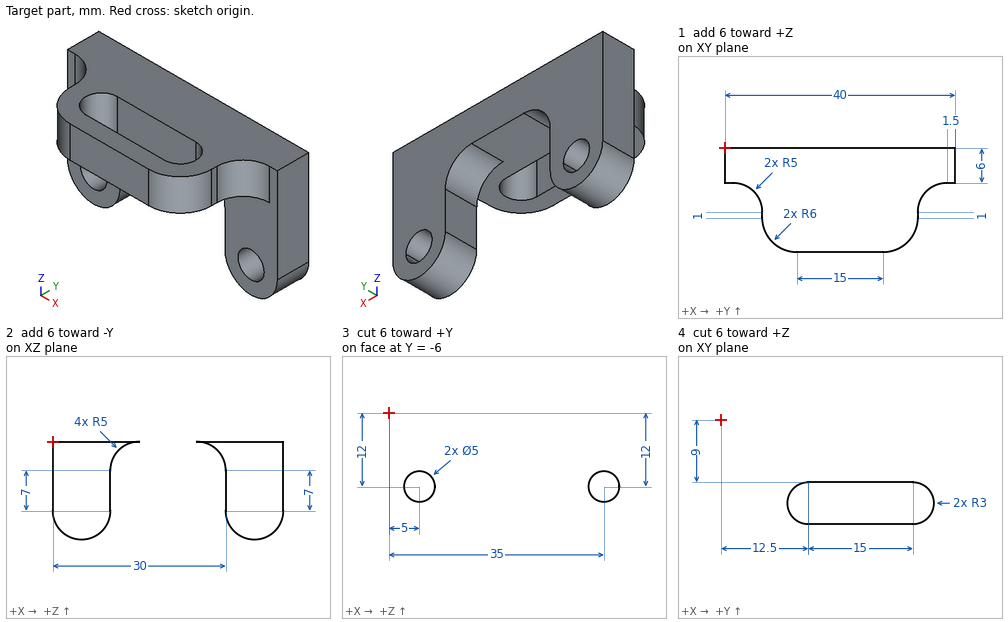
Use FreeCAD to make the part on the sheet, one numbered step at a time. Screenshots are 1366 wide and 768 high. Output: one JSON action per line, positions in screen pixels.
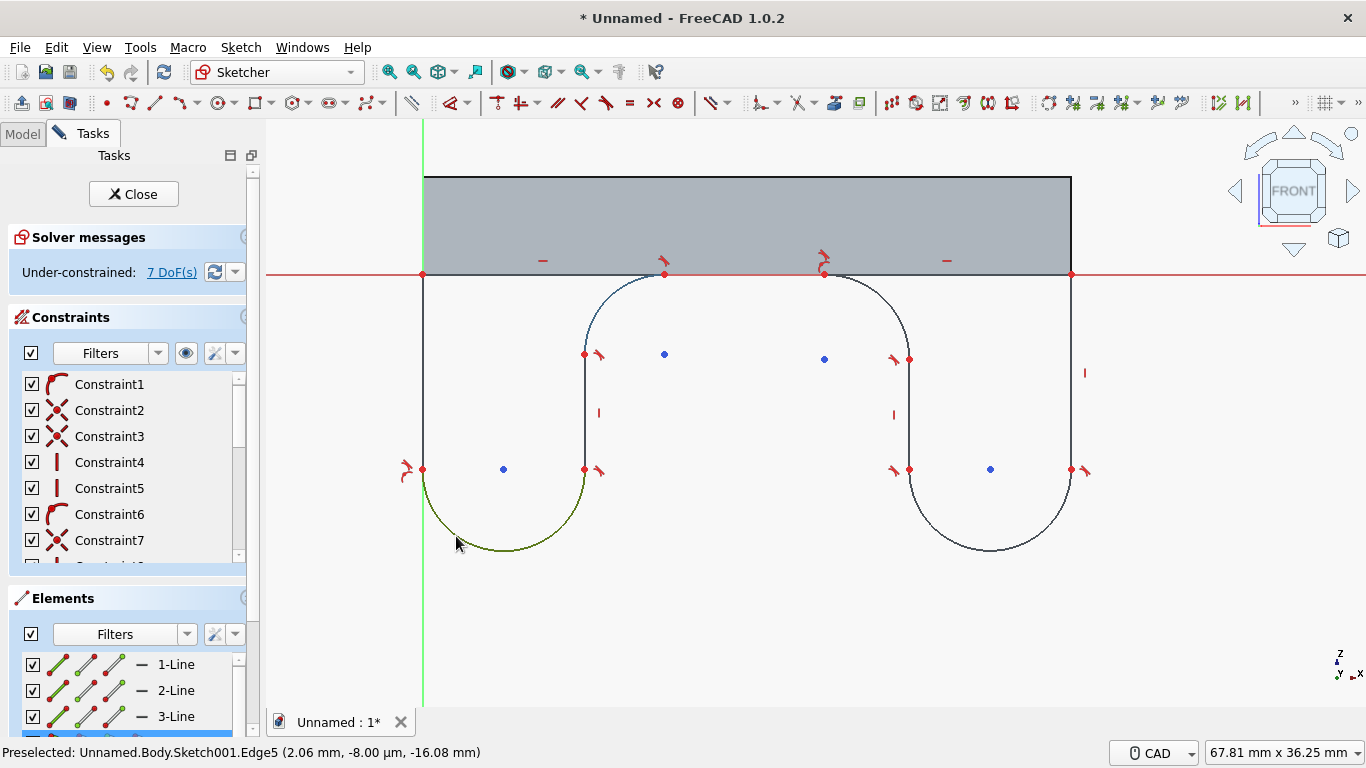
{"action": "left_click", "coordinate": [900, 321]}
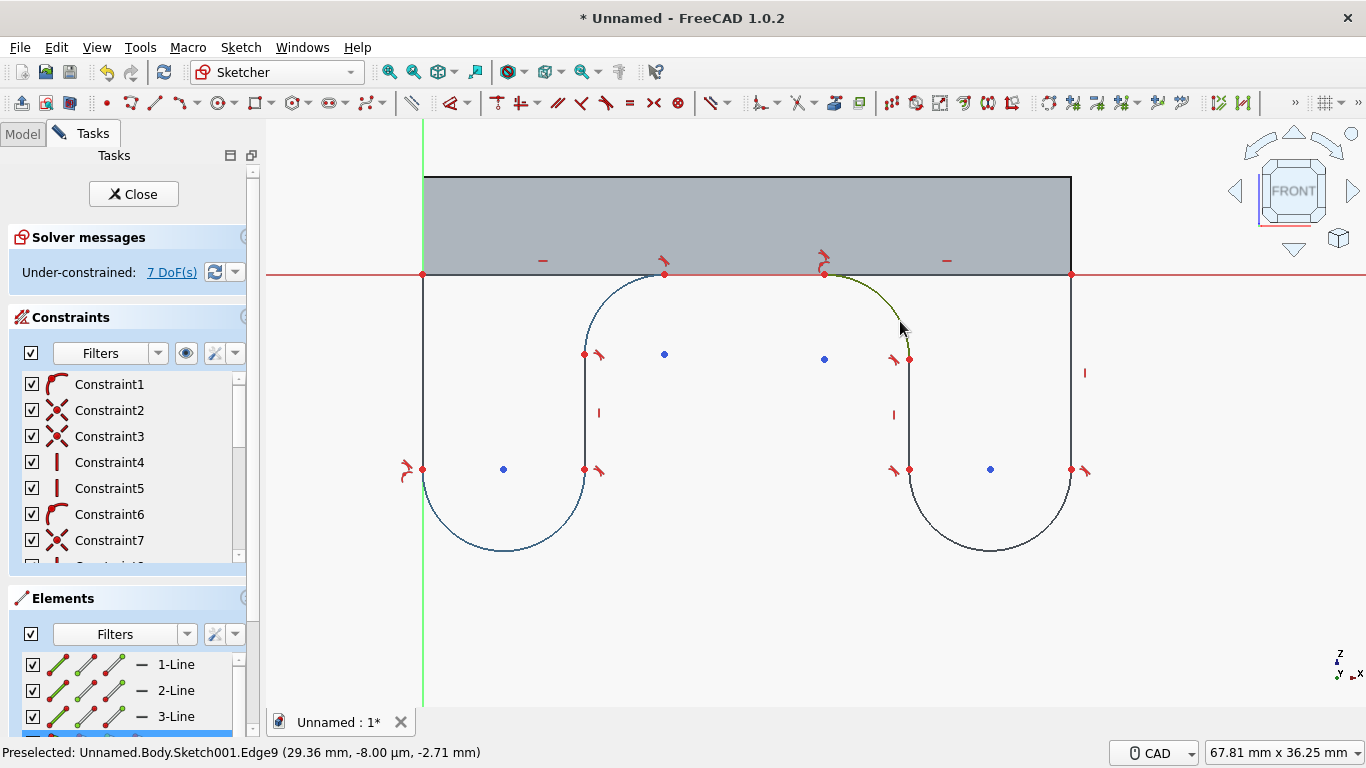
{"action": "left_click", "coordinate": [943, 535]}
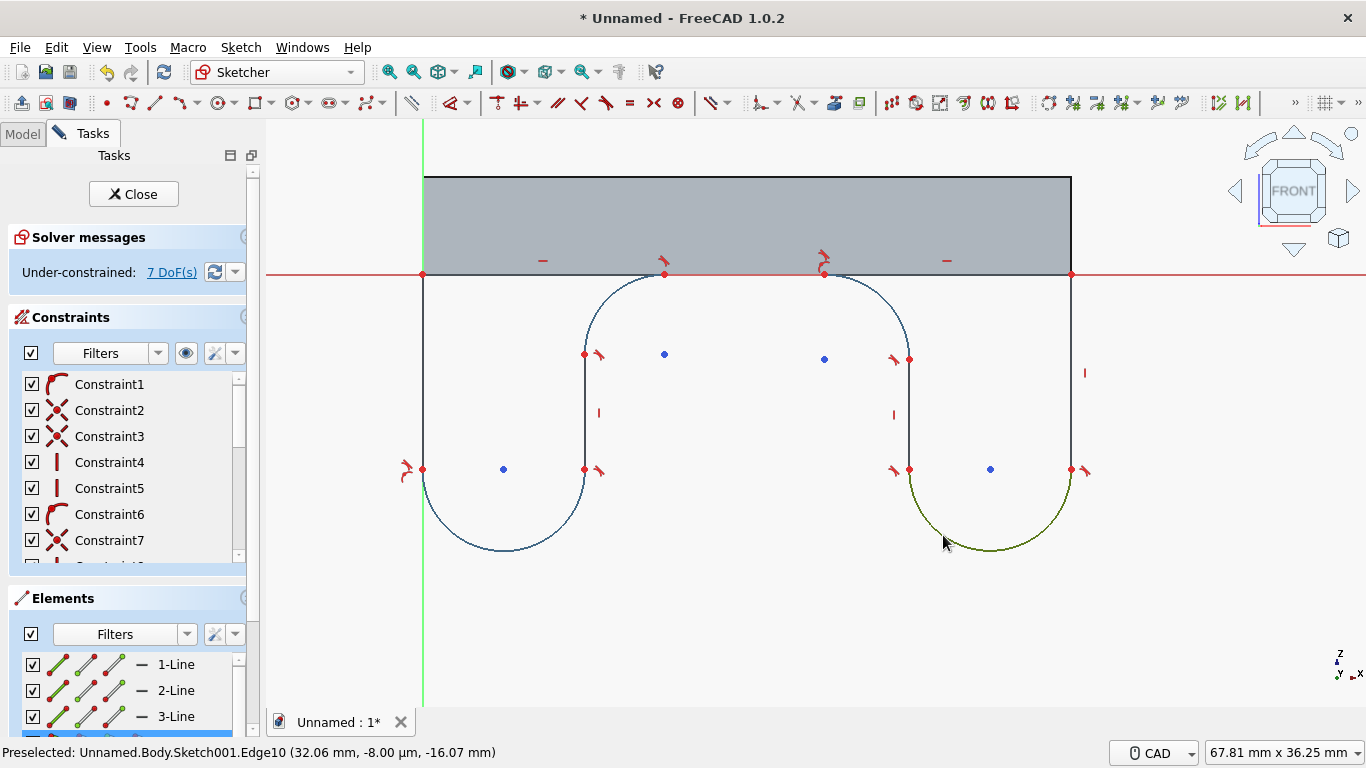
{"action": "key", "text": "e"}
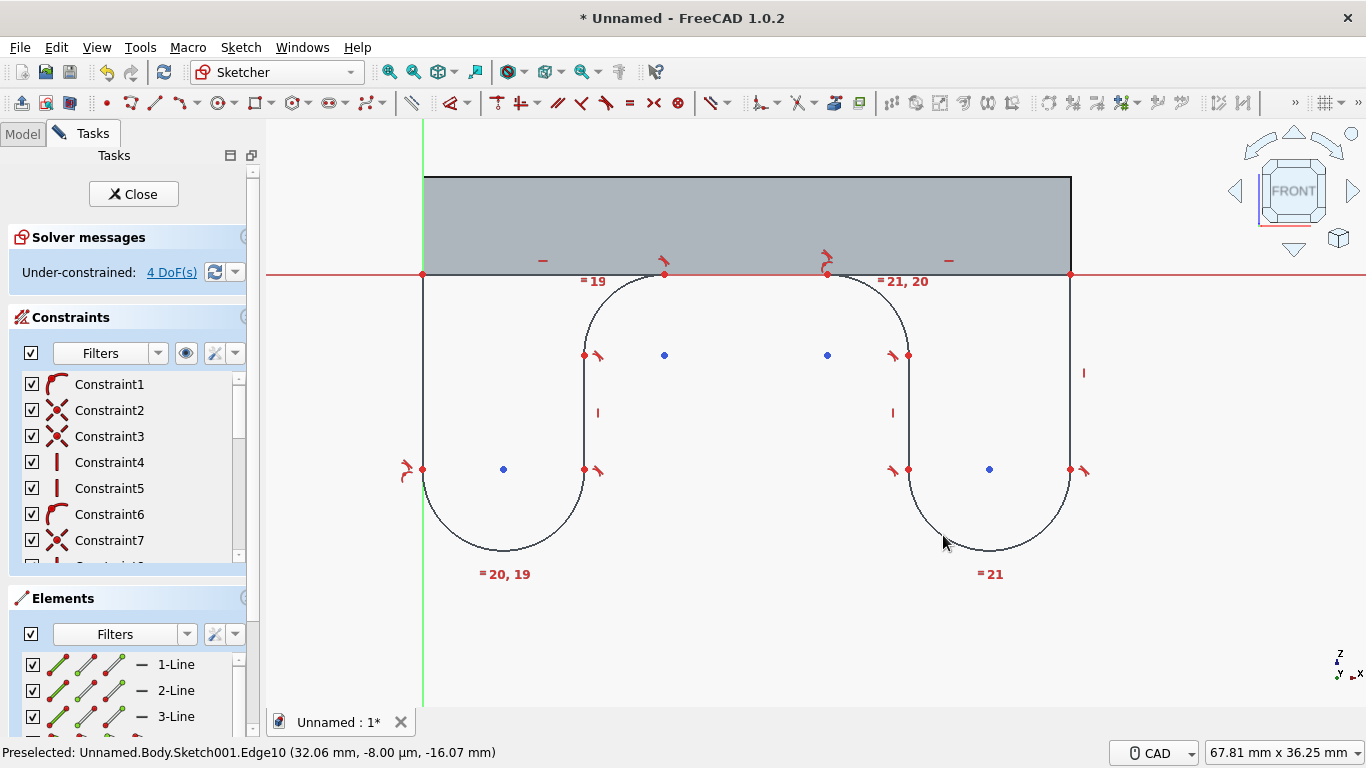
{"action": "key", "text": "d"}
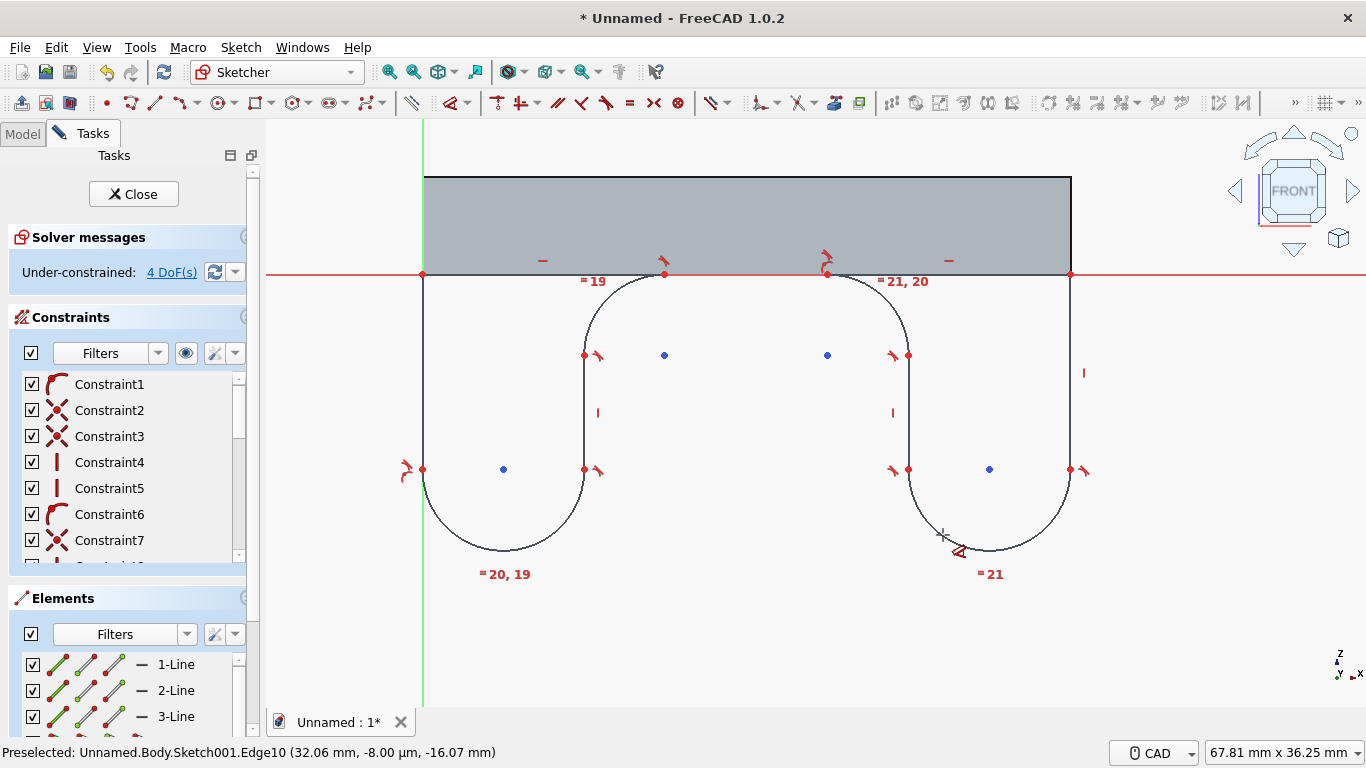
{"action": "left_click", "coordinate": [593, 319]}
{"action": "left_click", "coordinate": [564, 305]}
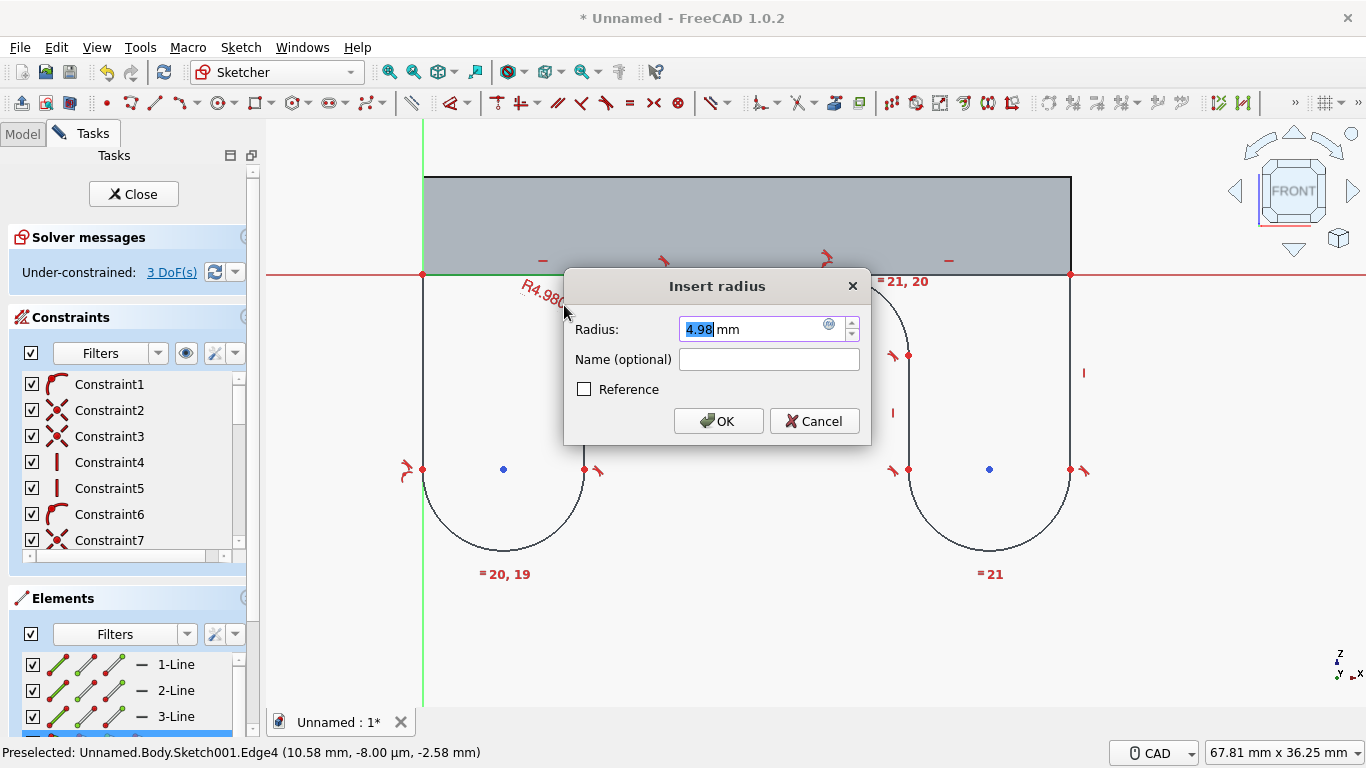
{"action": "type", "text": "5"}
{"action": "key", "text": "Return"}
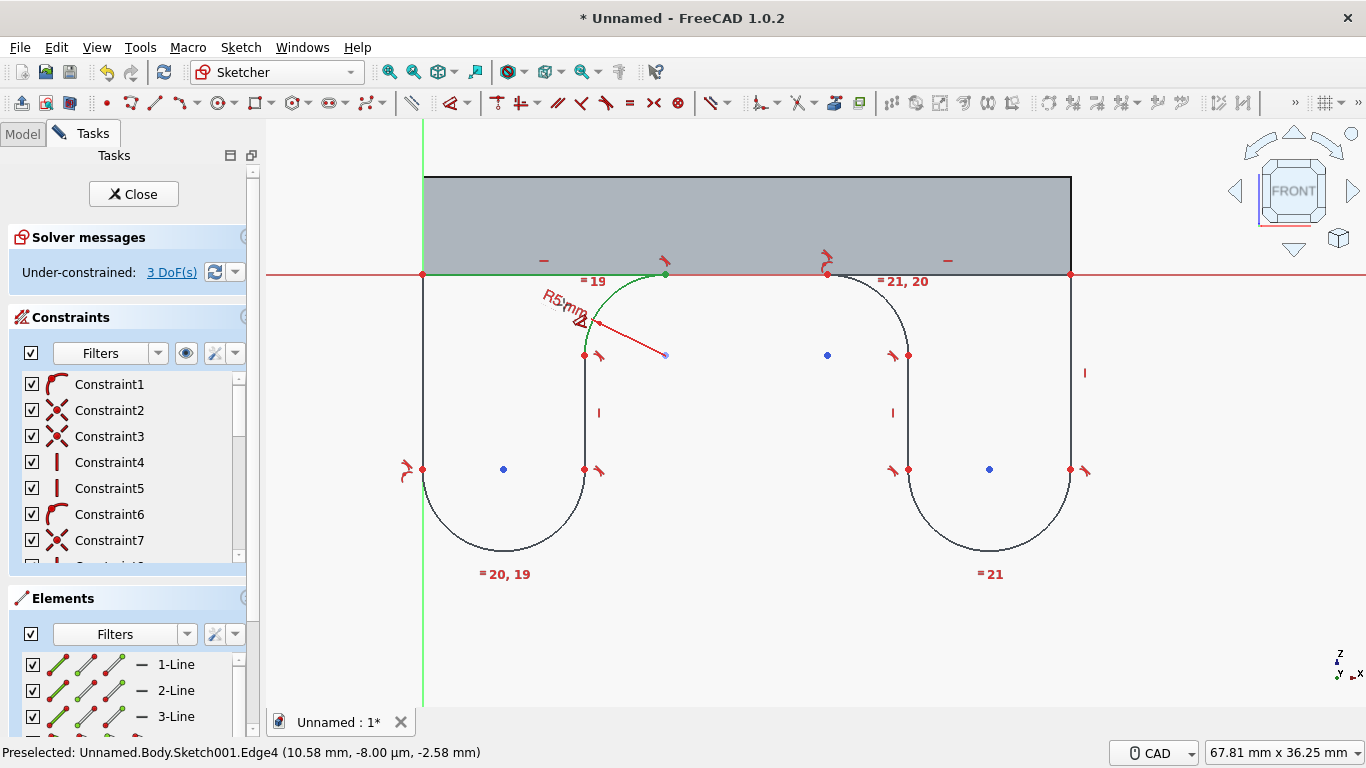
{"action": "left_click", "coordinate": [585, 390]}
{"action": "left_click", "coordinate": [551, 413]}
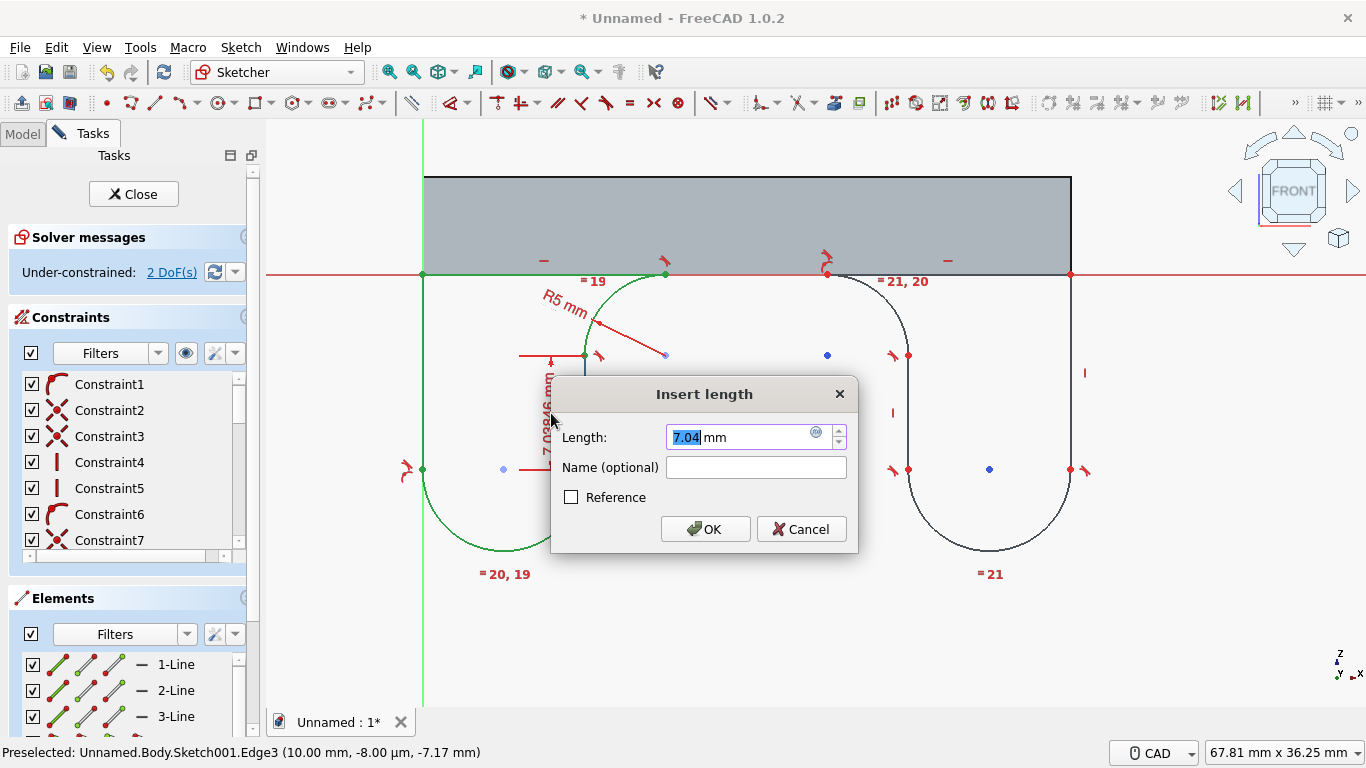
{"action": "type", "text": "7"}
{"action": "key", "text": "Return"}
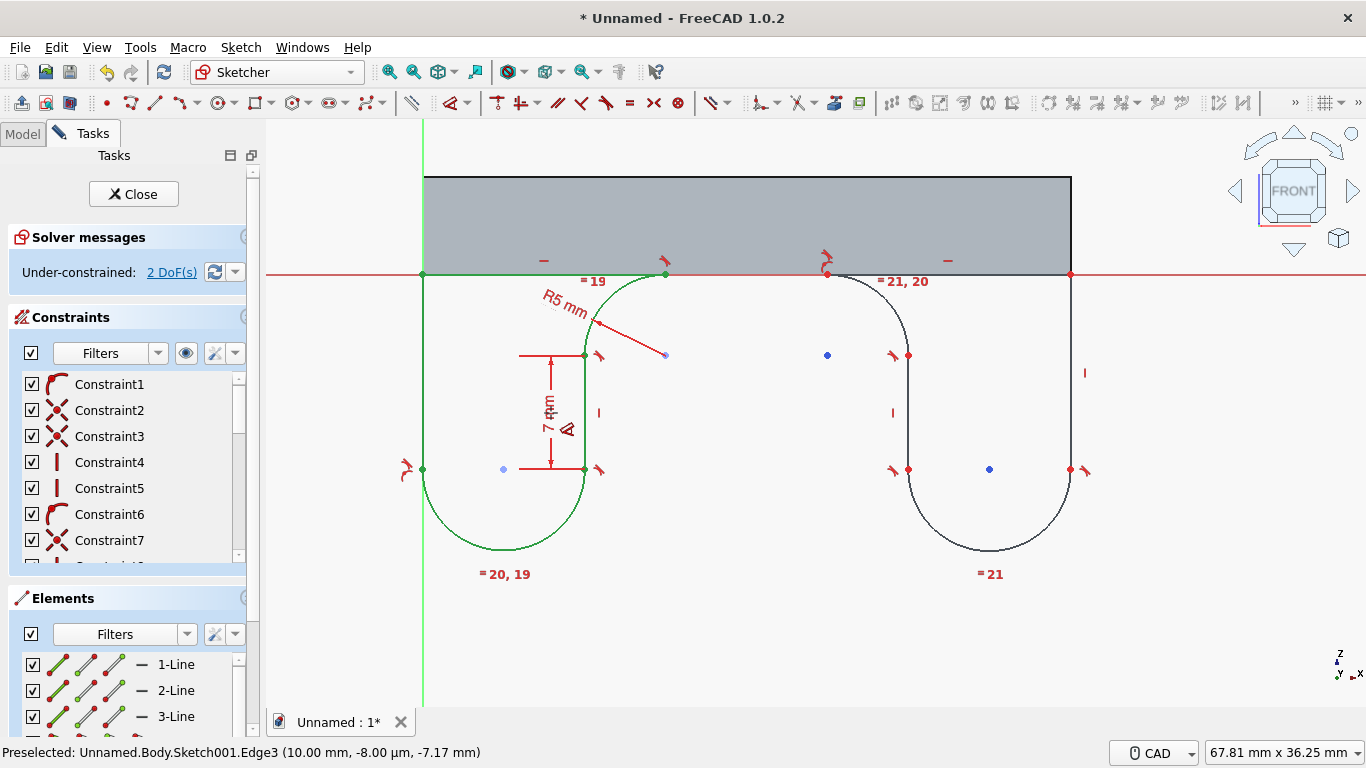
{"action": "left_click", "coordinate": [908, 436]}
{"action": "left_click", "coordinate": [942, 413]}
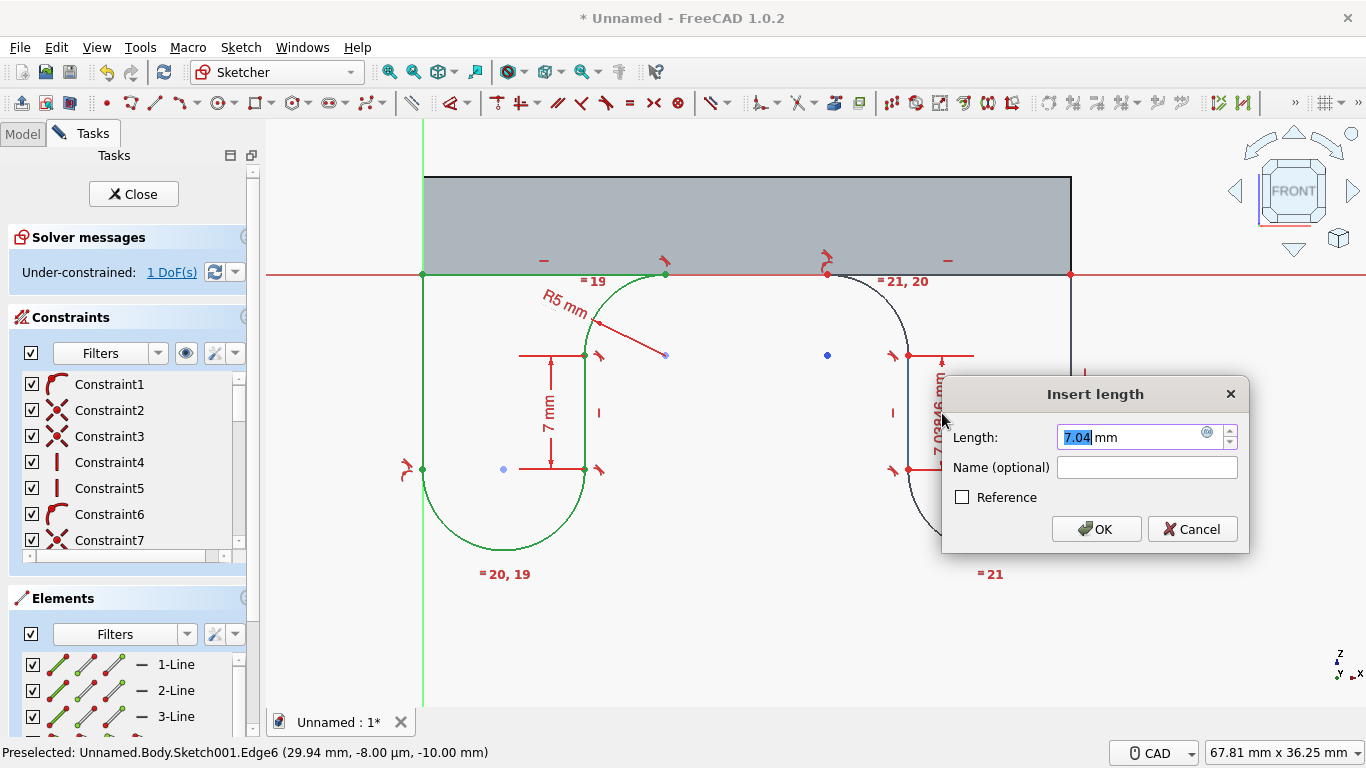
{"action": "type", "text": "7"}
{"action": "key", "text": "Return"}